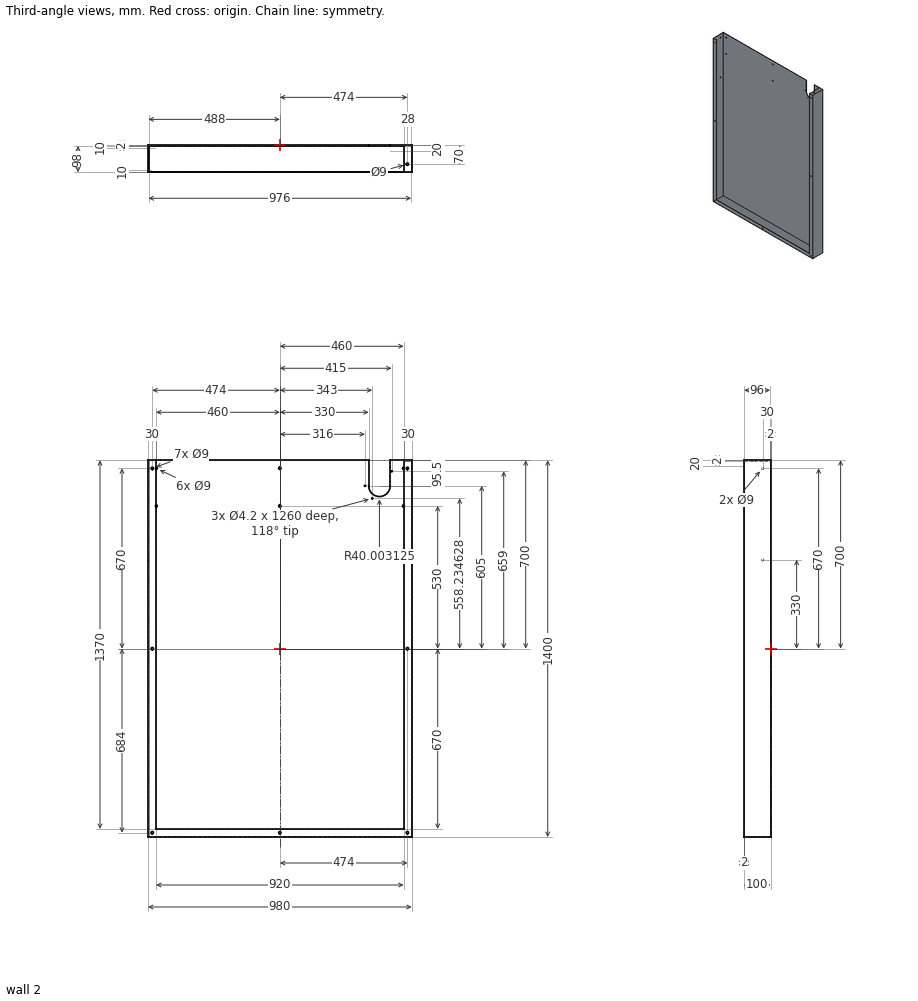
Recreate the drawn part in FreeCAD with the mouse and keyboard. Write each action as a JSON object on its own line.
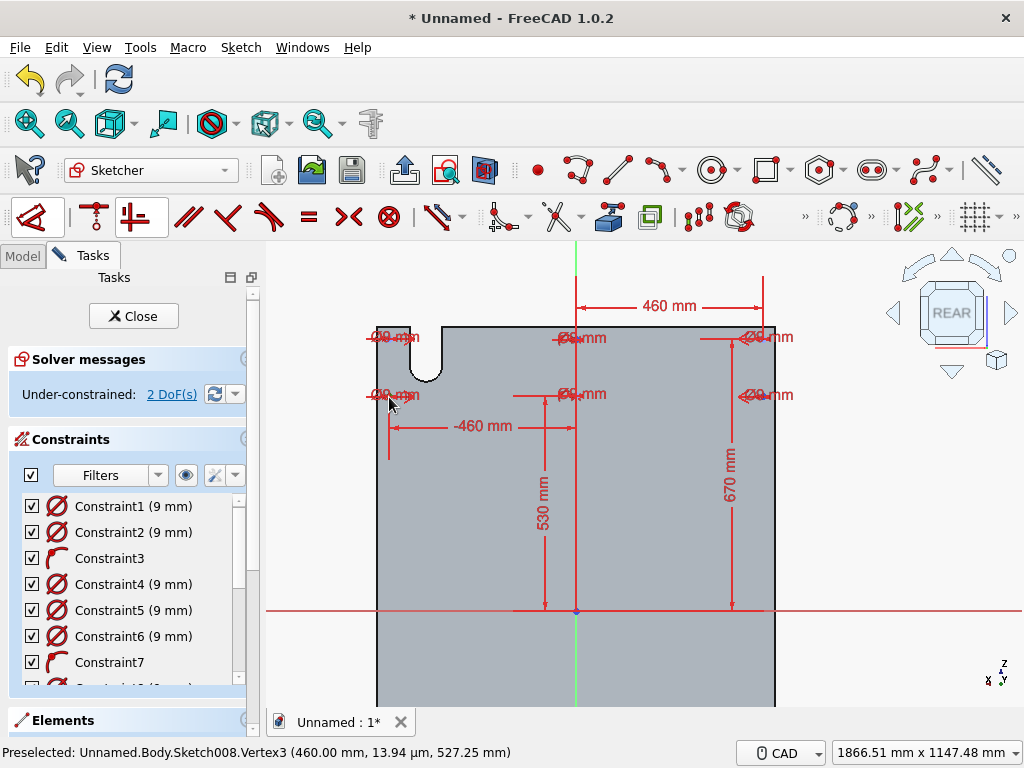
{"action": "left_click", "coordinate": [58, 218]}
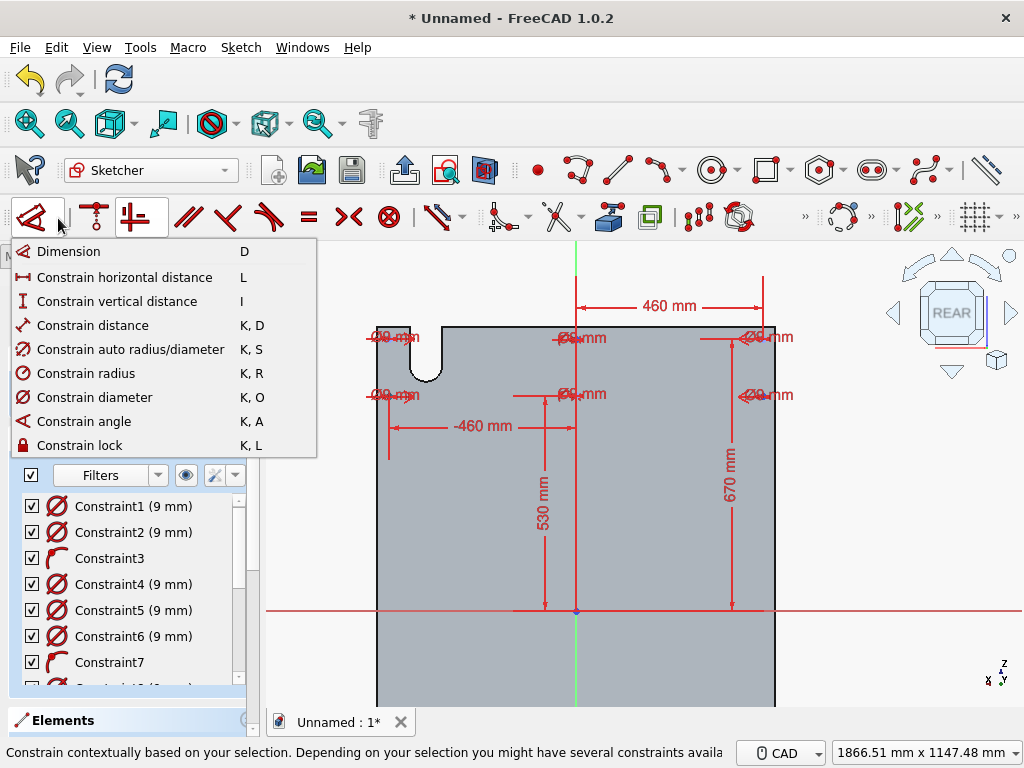
{"action": "left_click", "coordinate": [164, 301]}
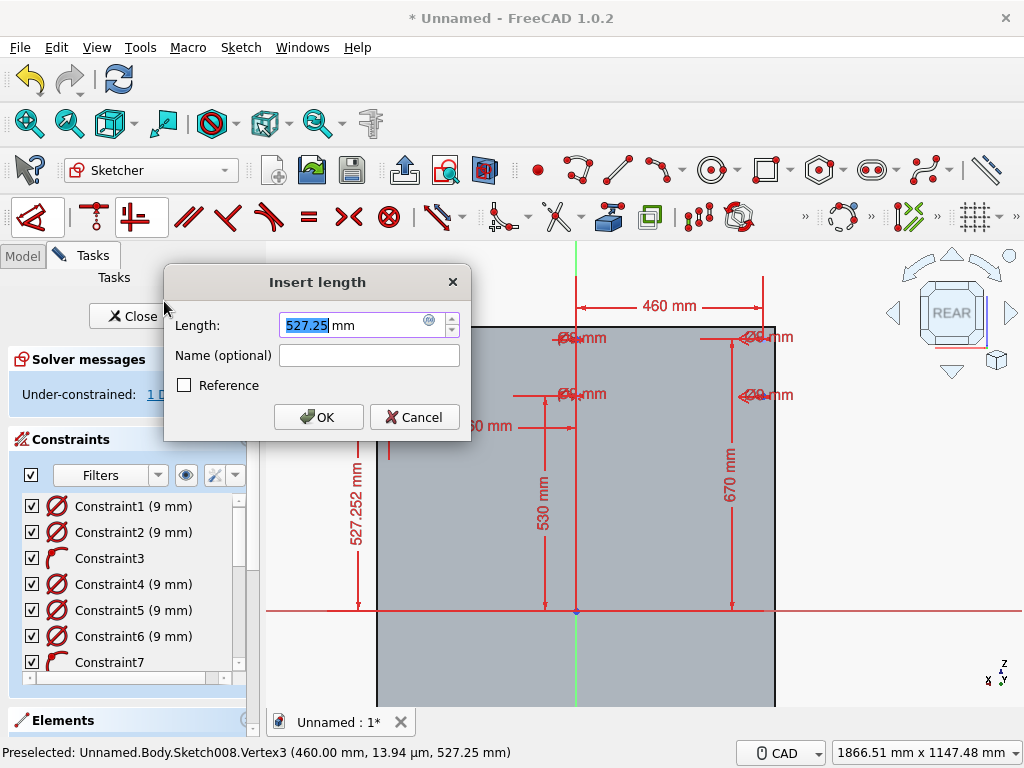
{"action": "type", "text": "530"}
{"action": "key", "text": "Return"}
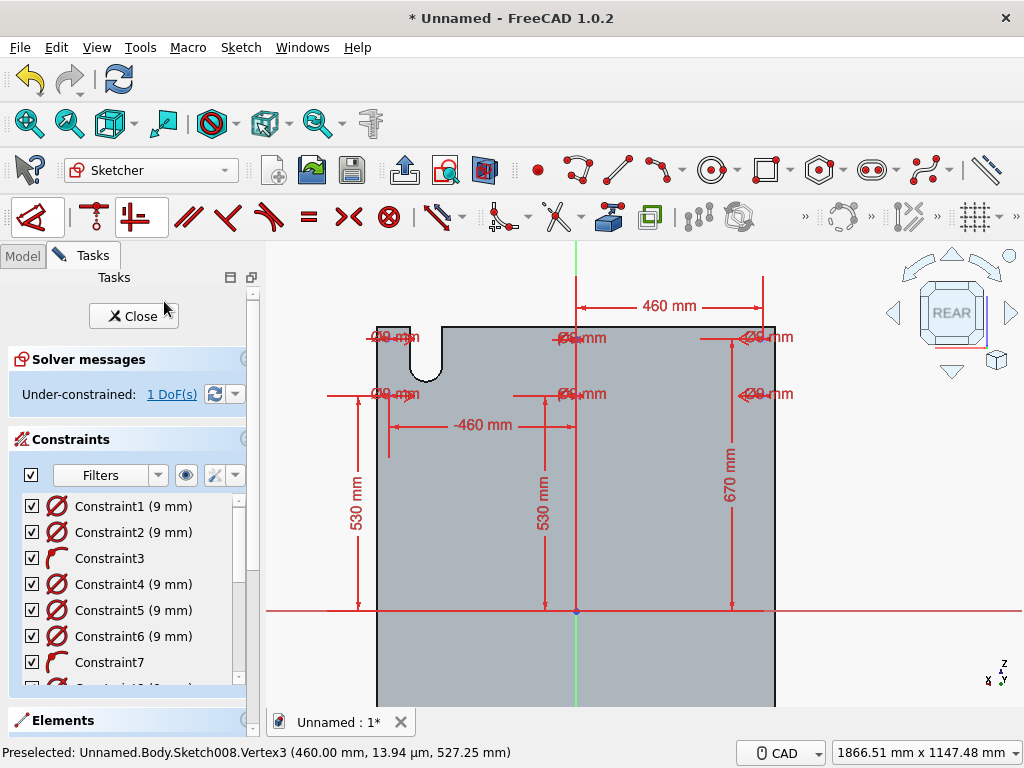
{"action": "left_click", "coordinate": [576, 340]}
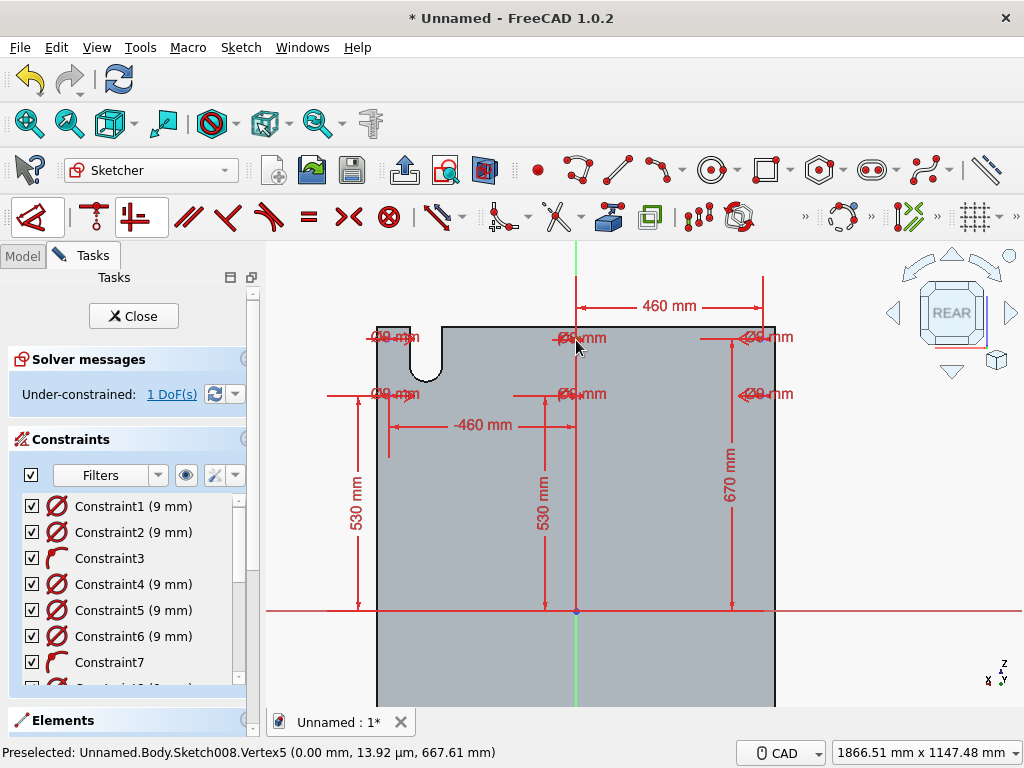
{"action": "left_click", "coordinate": [58, 218]}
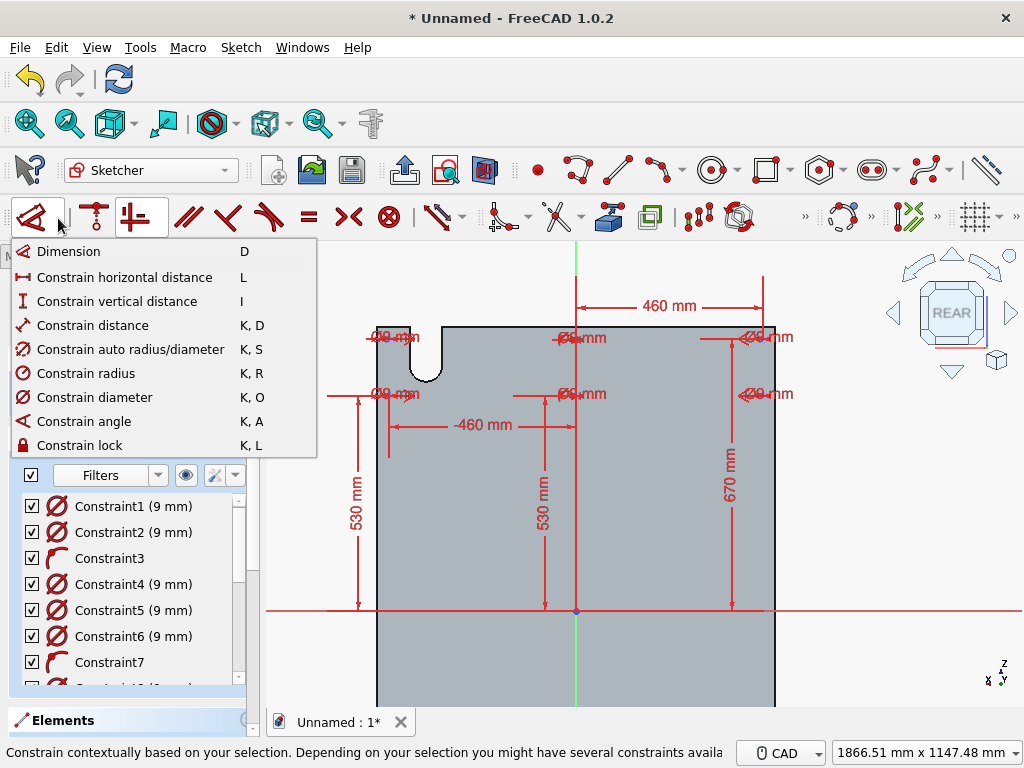
{"action": "left_click", "coordinate": [164, 301]}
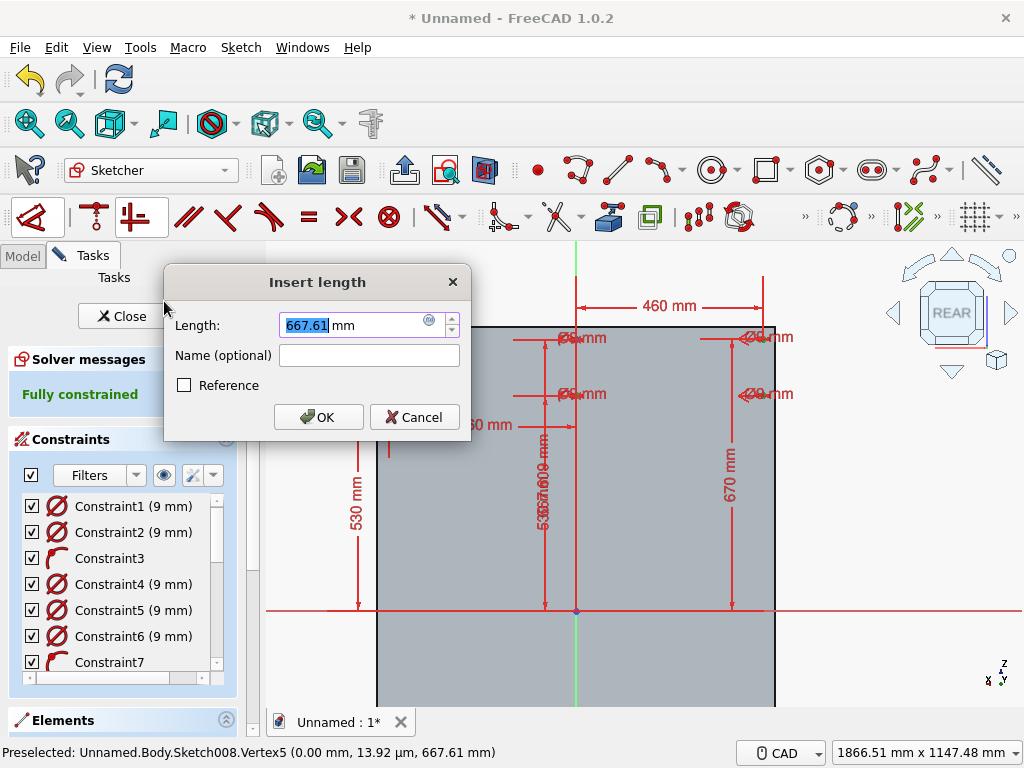
{"action": "type", "text": "670"}
{"action": "key", "text": "Return"}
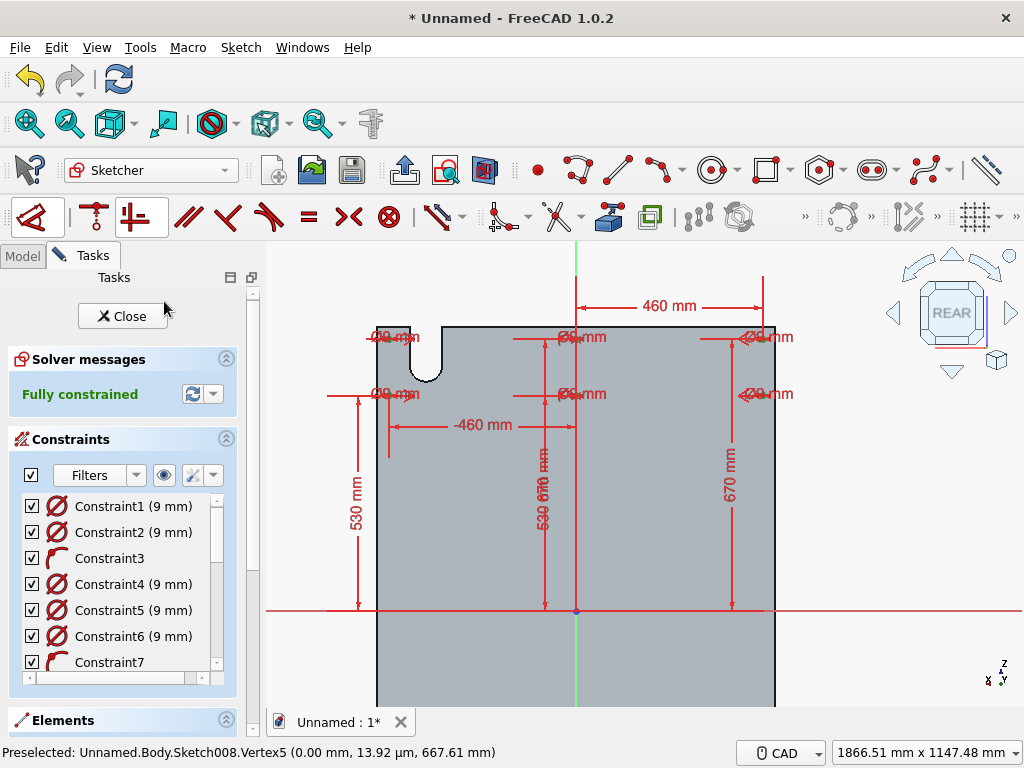
{"action": "left_click", "coordinate": [123, 316]}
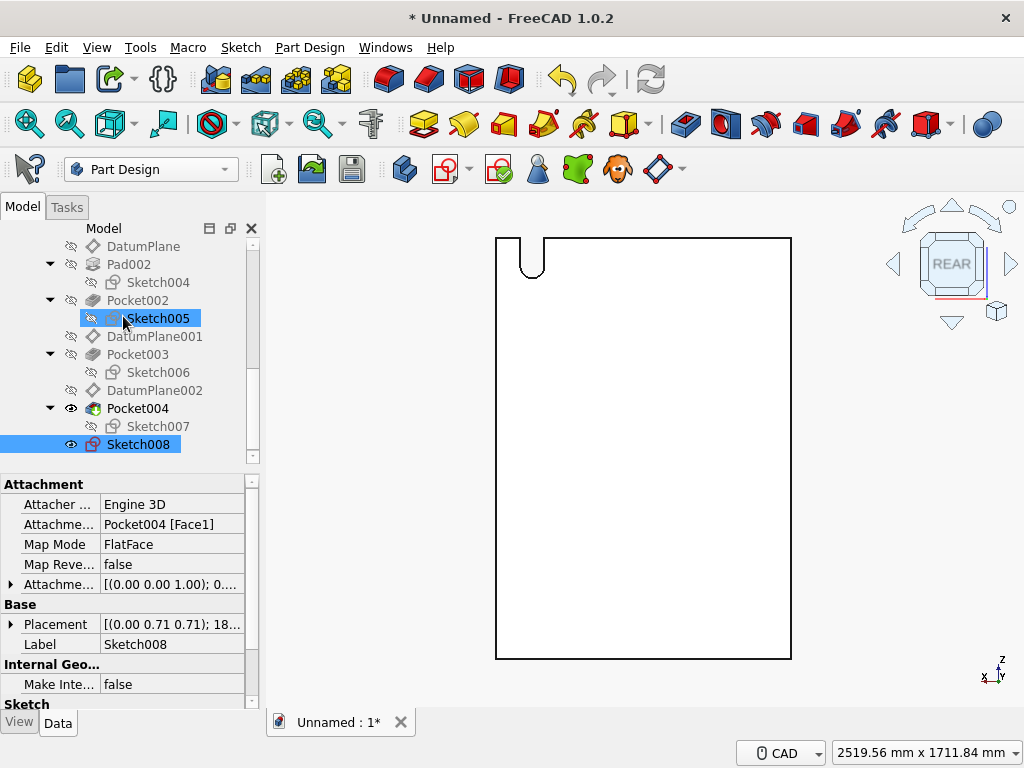
{"action": "left_click", "coordinate": [686, 124]}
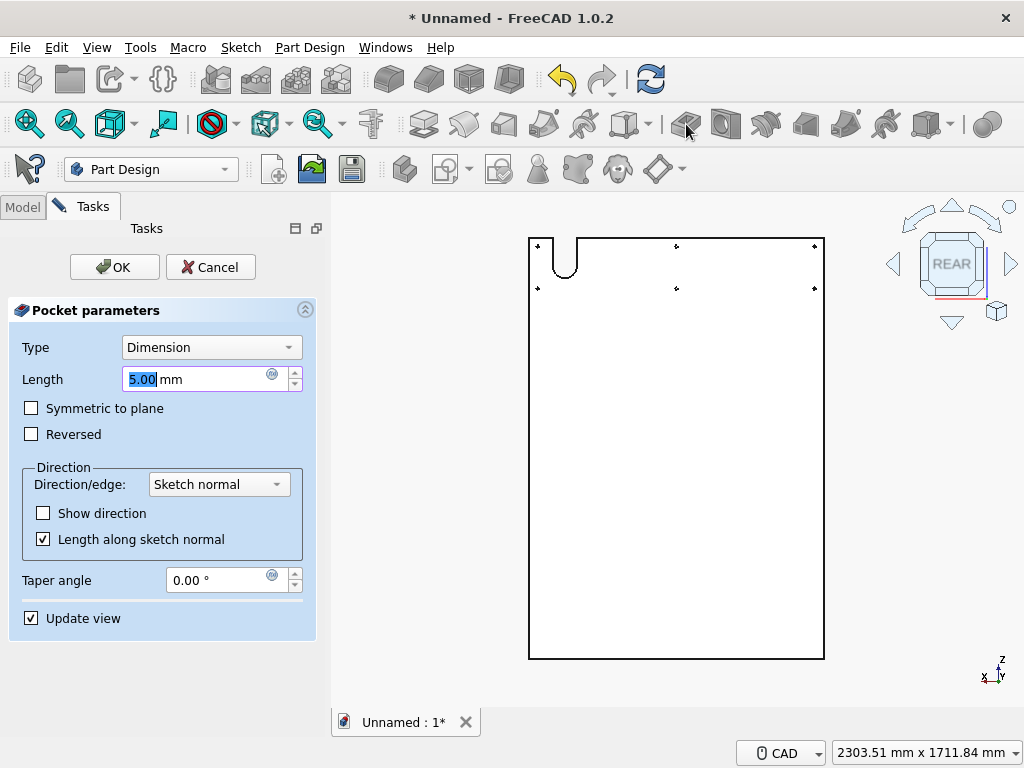
{"action": "type", "text": "10"}
{"action": "key", "text": "Tab"}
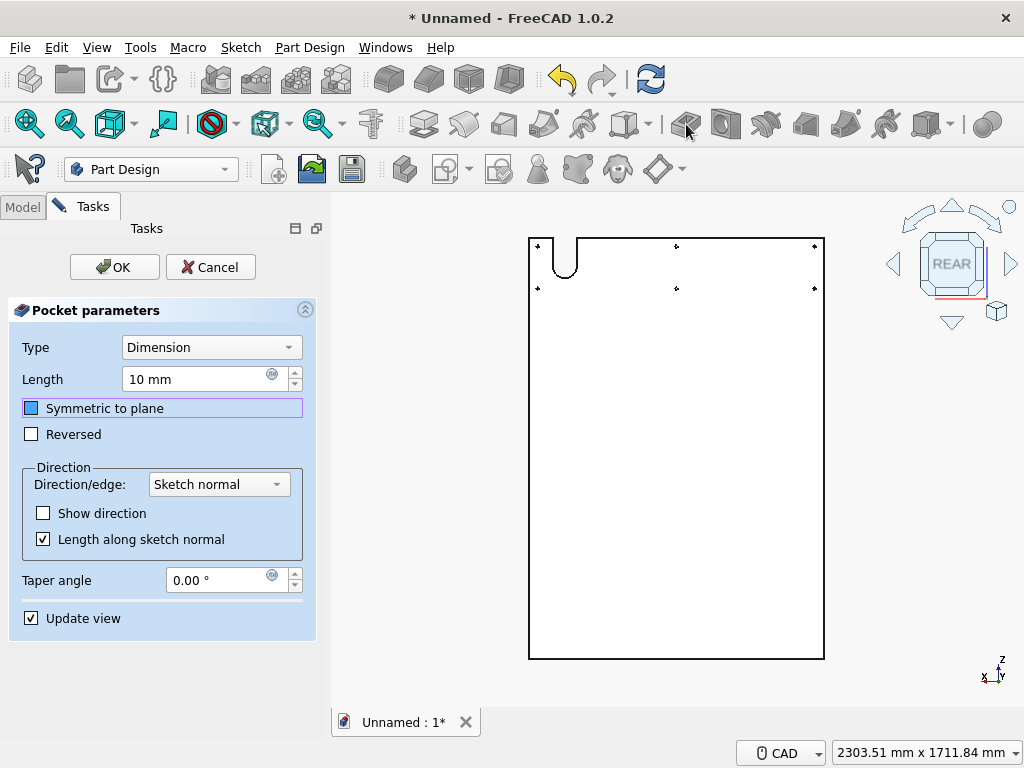
{"action": "left_click", "coordinate": [115, 267]}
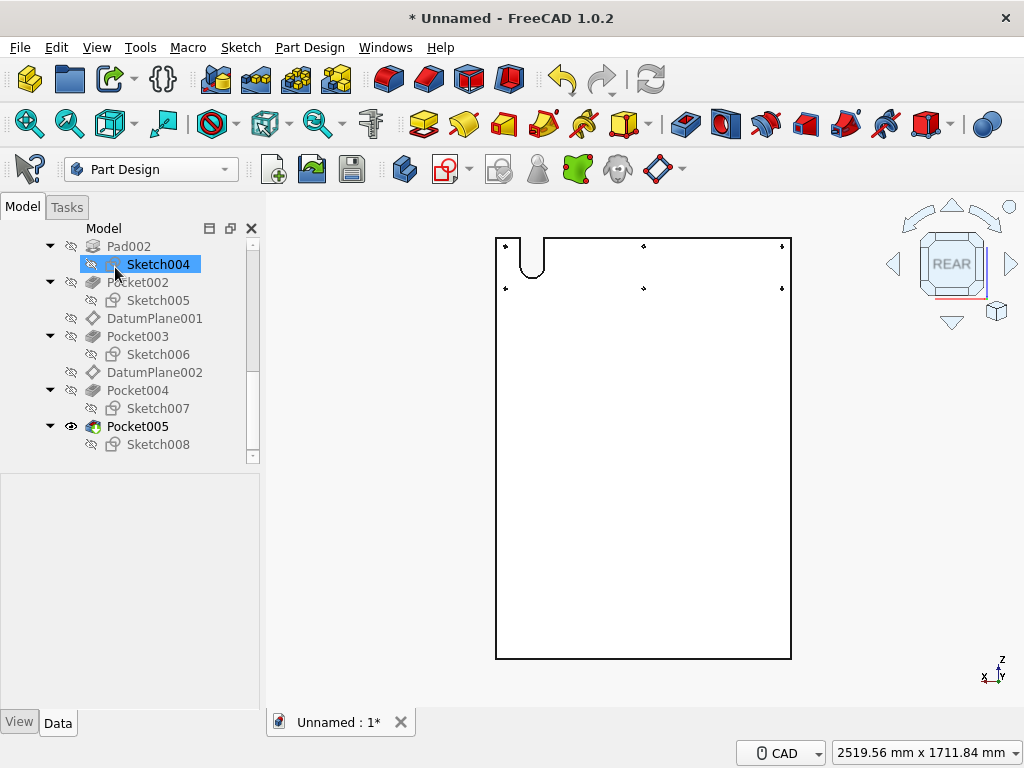
{"action": "left_click", "coordinate": [446, 170]}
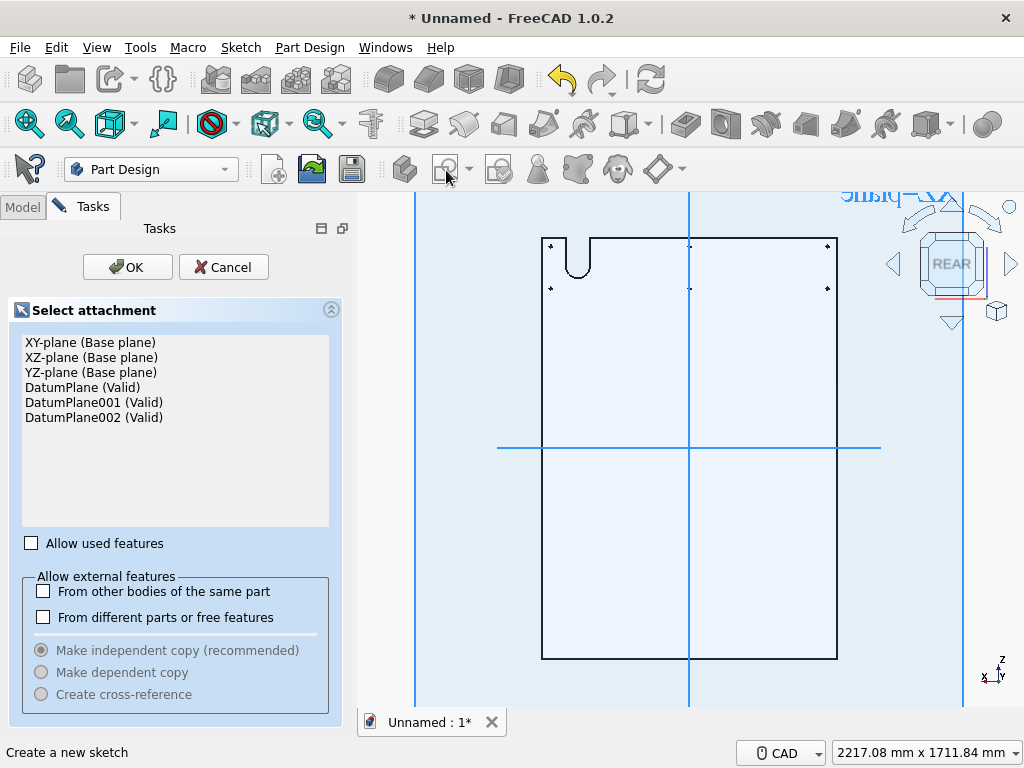
{"action": "left_click", "coordinate": [82, 358]}